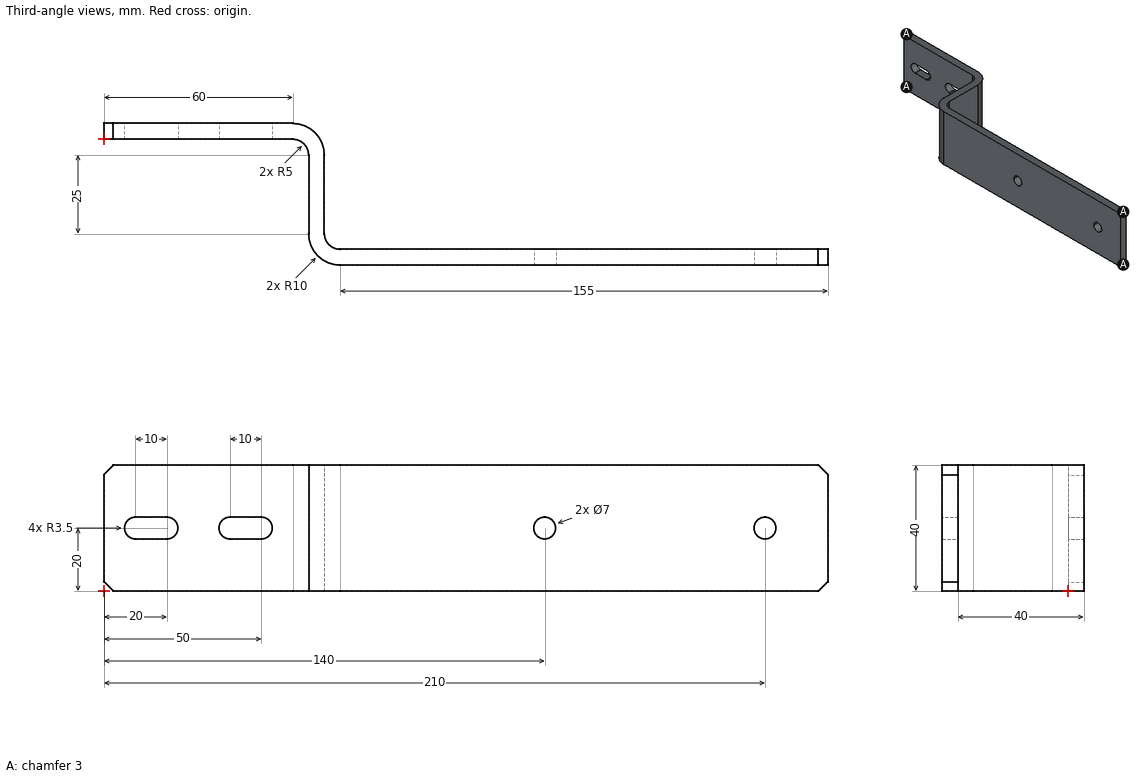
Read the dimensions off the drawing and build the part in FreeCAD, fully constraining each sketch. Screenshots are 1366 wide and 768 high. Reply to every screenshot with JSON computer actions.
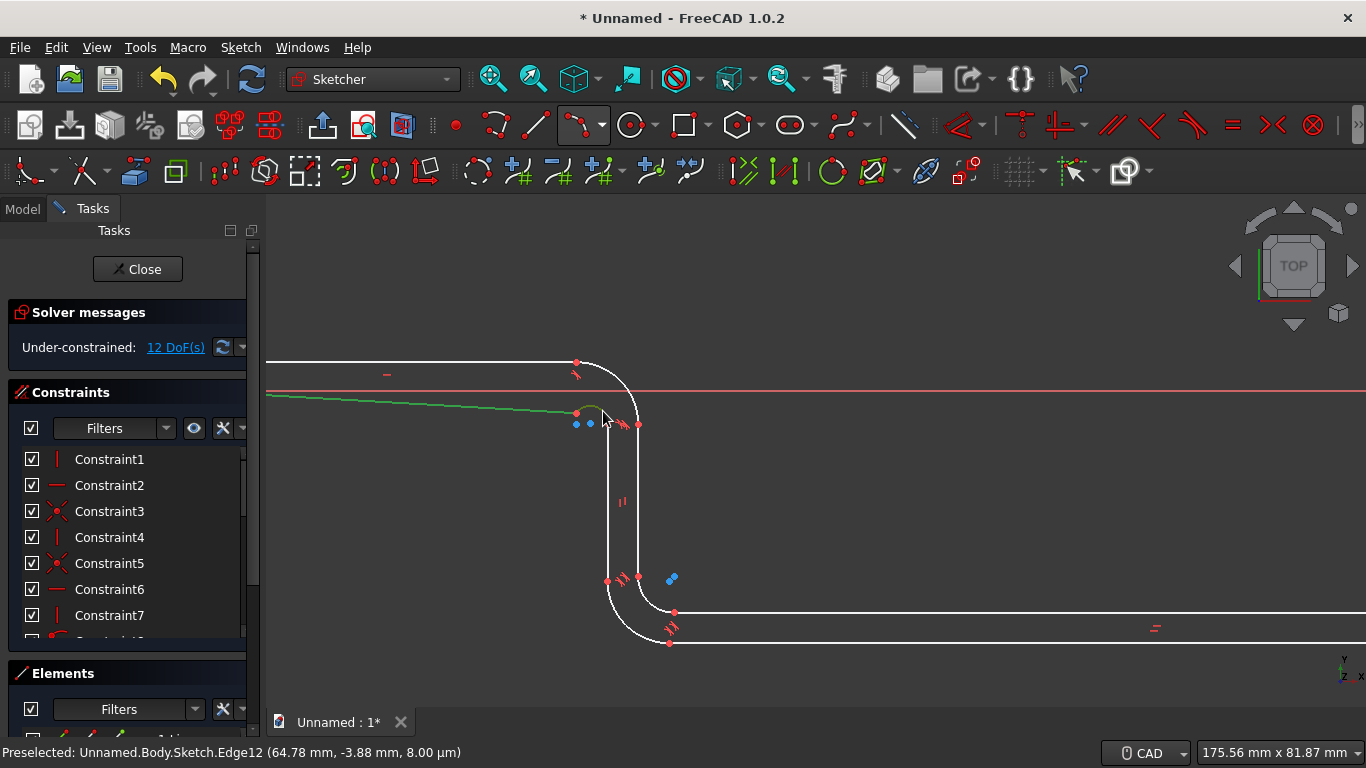
{"action": "left_click", "coordinate": [1194, 126]}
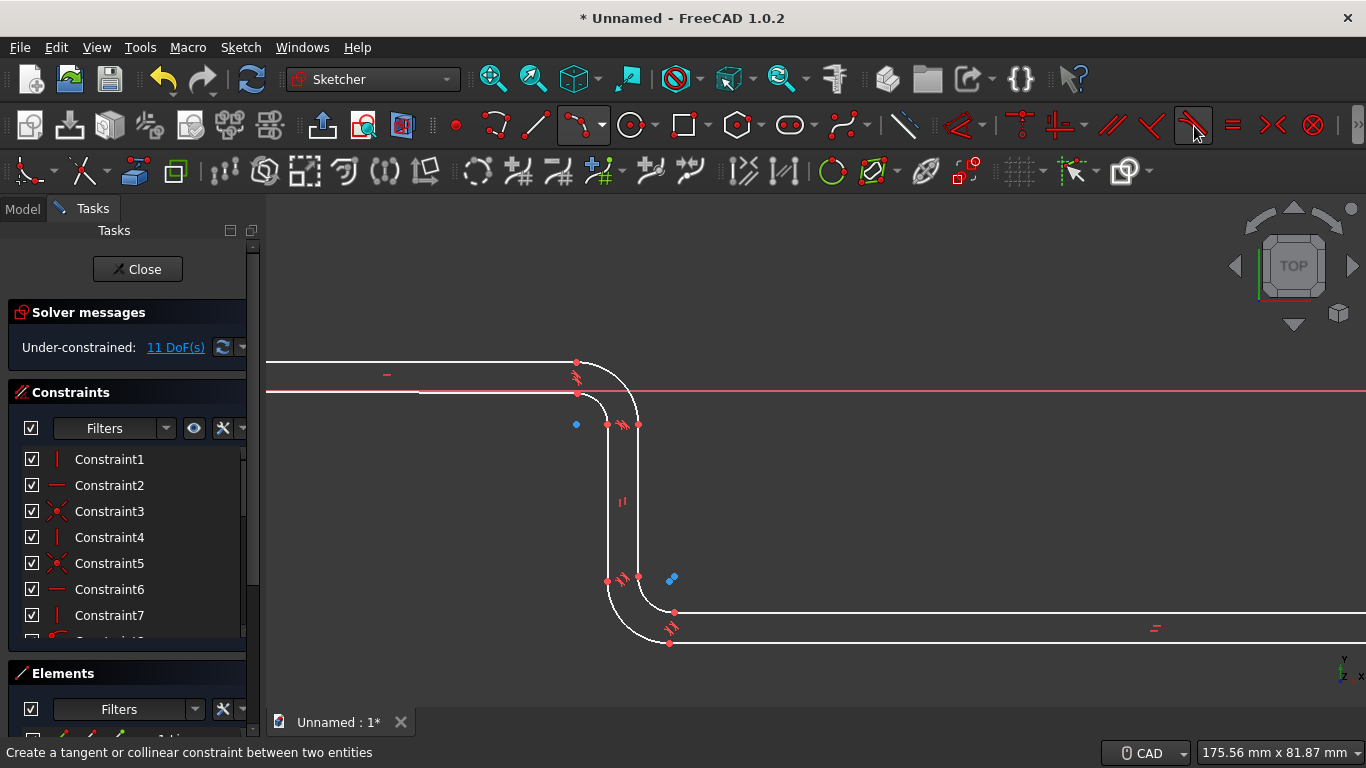
{"action": "left_click", "coordinate": [313, 392]}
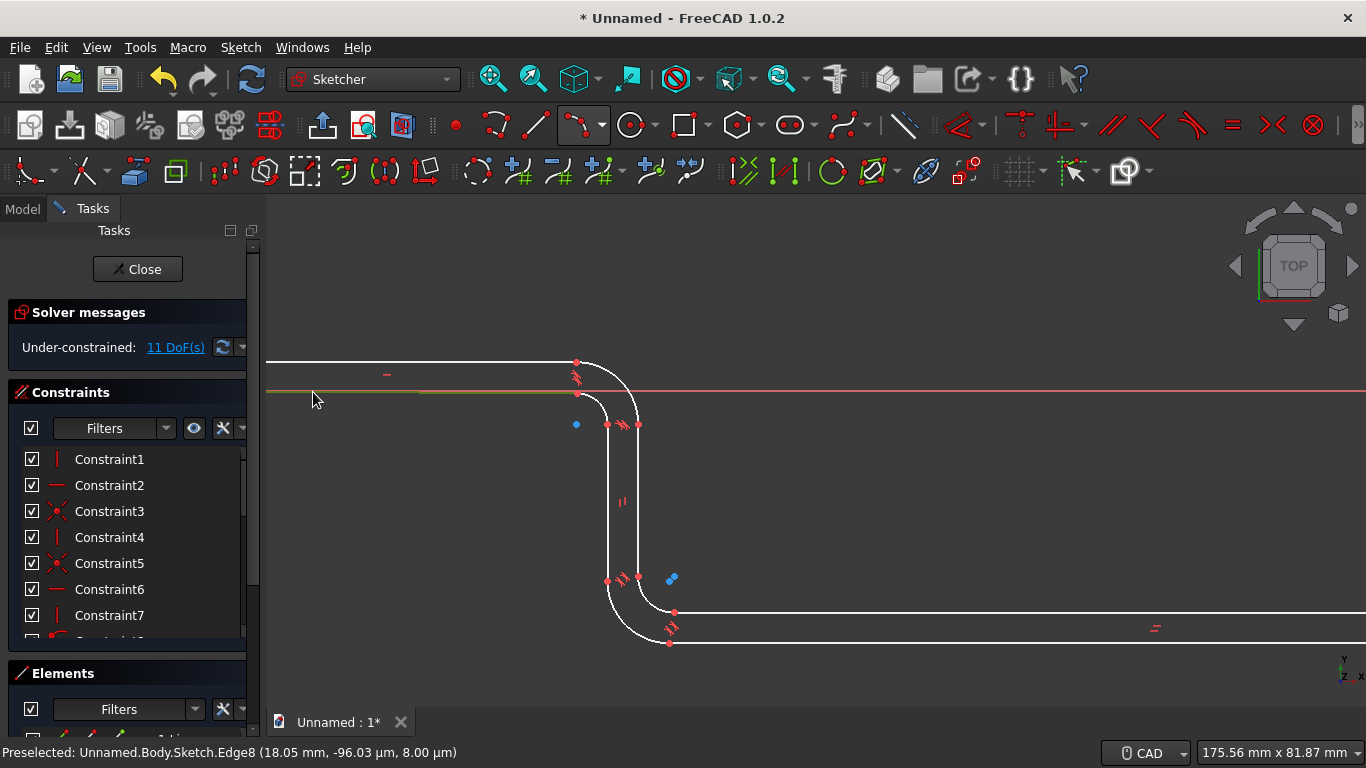
{"action": "key", "text": "h"}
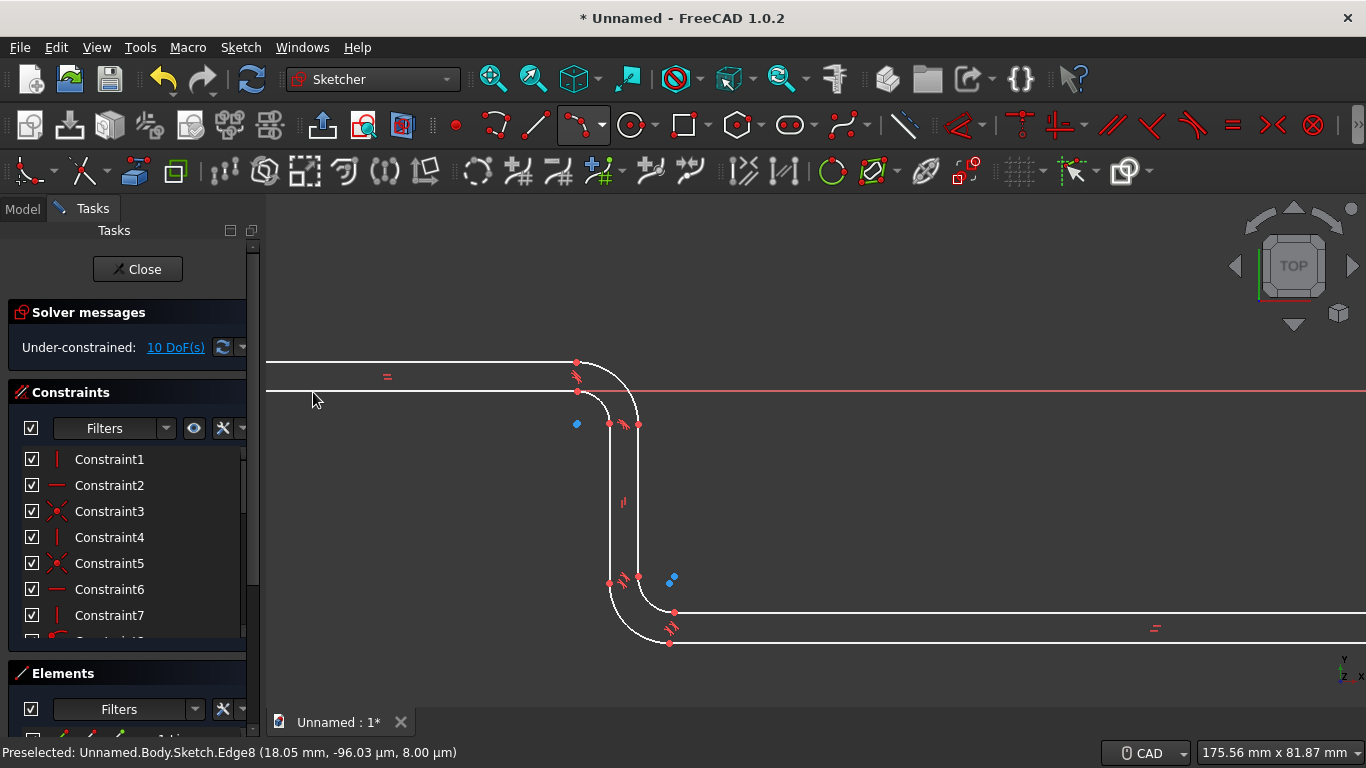
{"action": "left_click", "coordinate": [616, 610]}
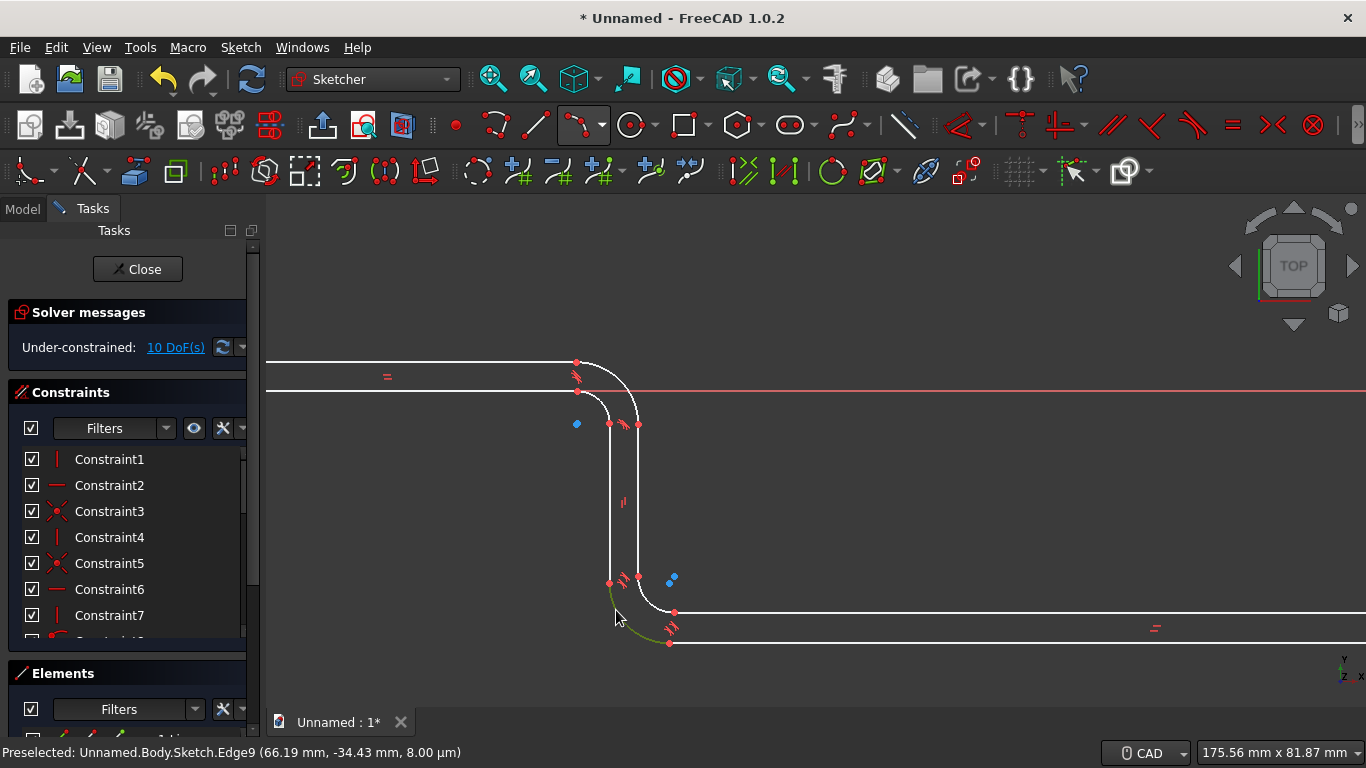
{"action": "left_click", "coordinate": [642, 593]}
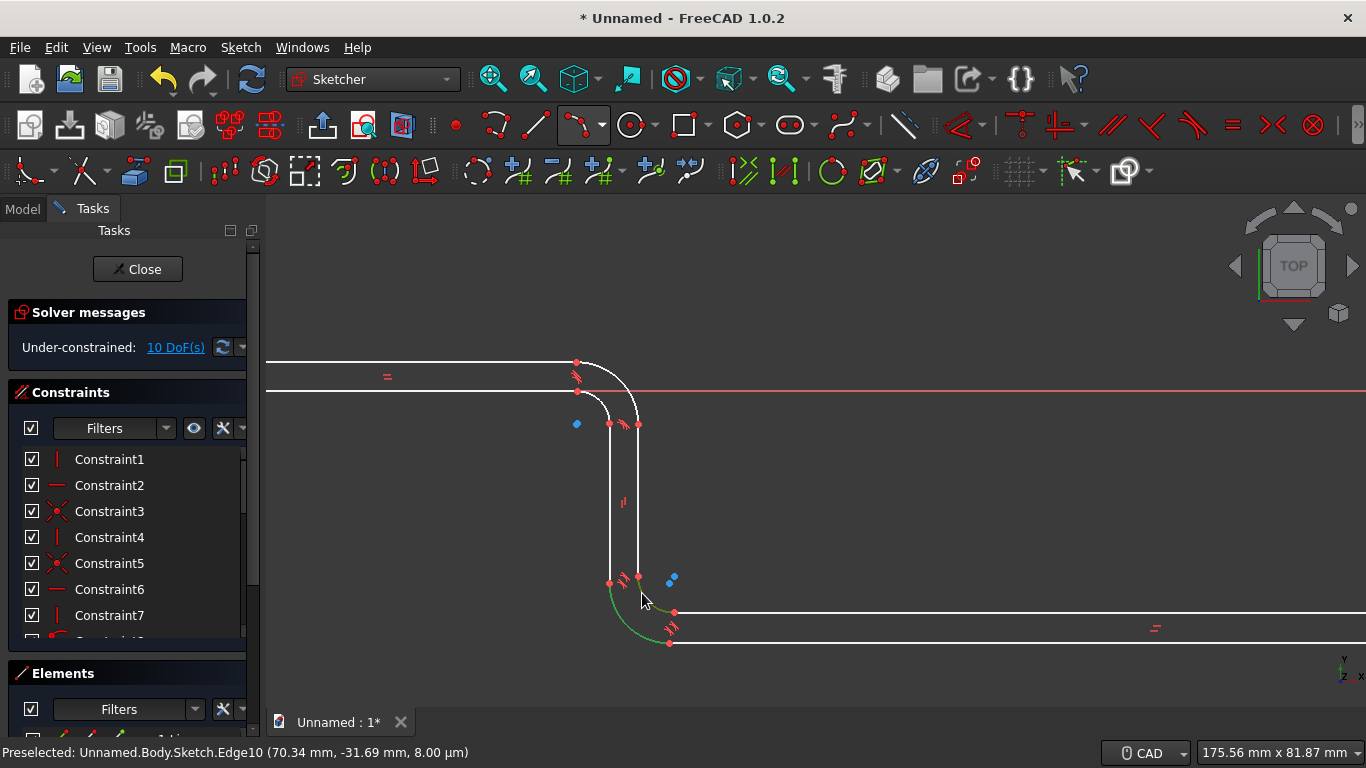
{"action": "left_click", "coordinate": [1020, 126]}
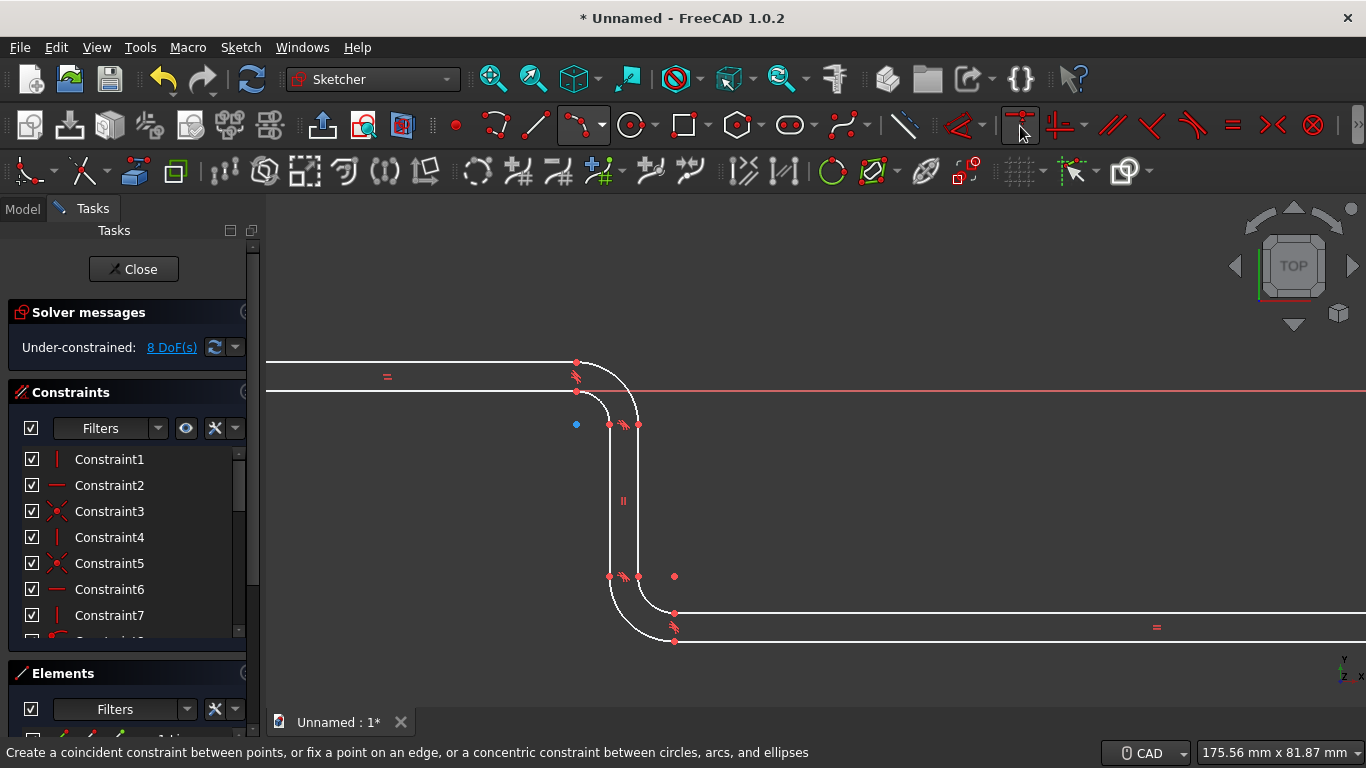
{"action": "left_click", "coordinate": [604, 369]}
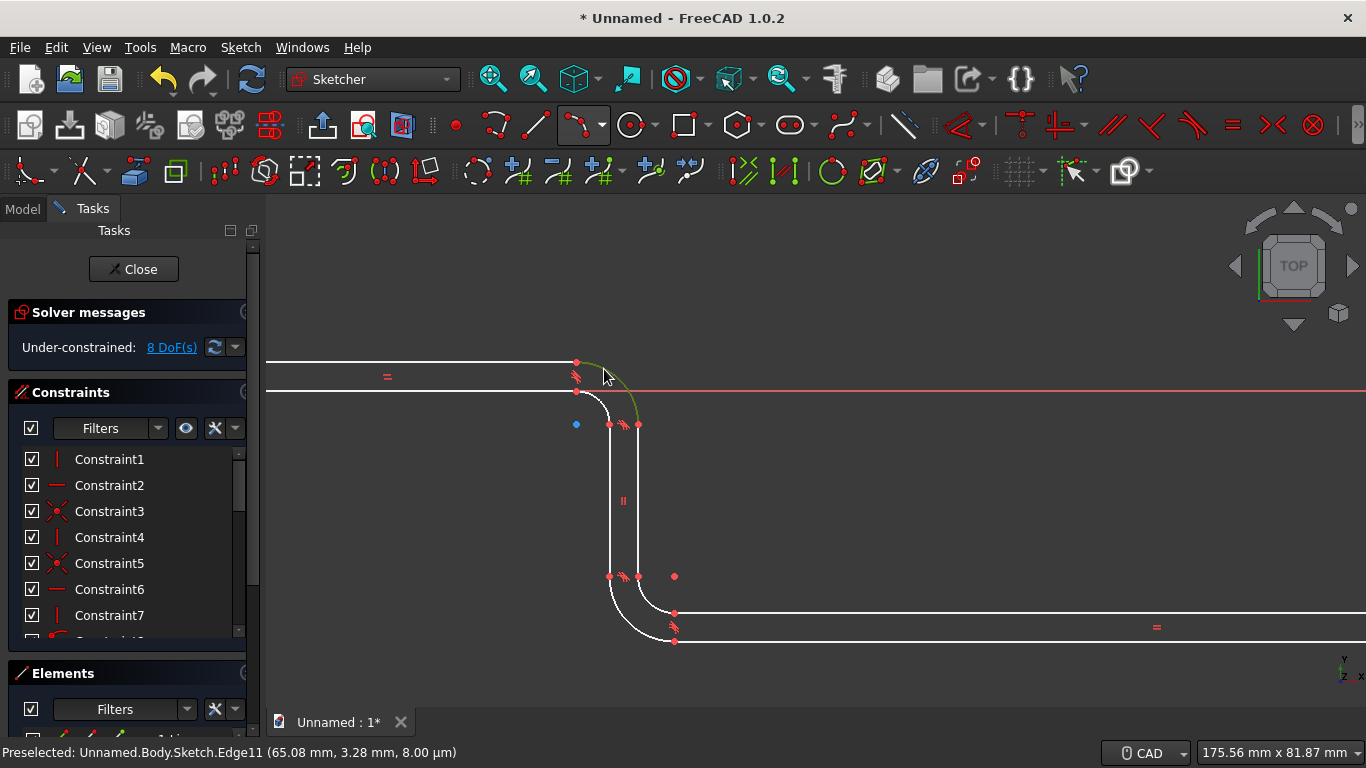
{"action": "left_click", "coordinate": [606, 409]}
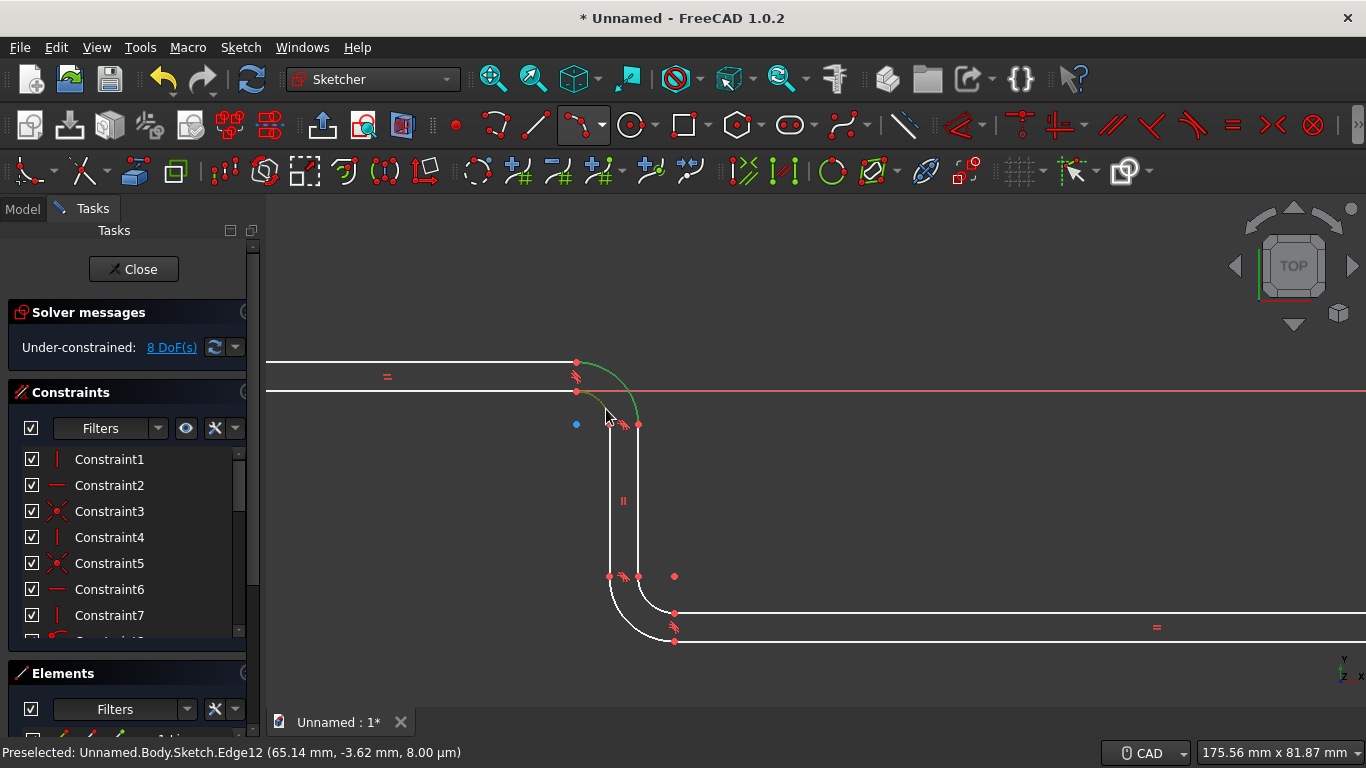
{"action": "left_click", "coordinate": [1020, 126]}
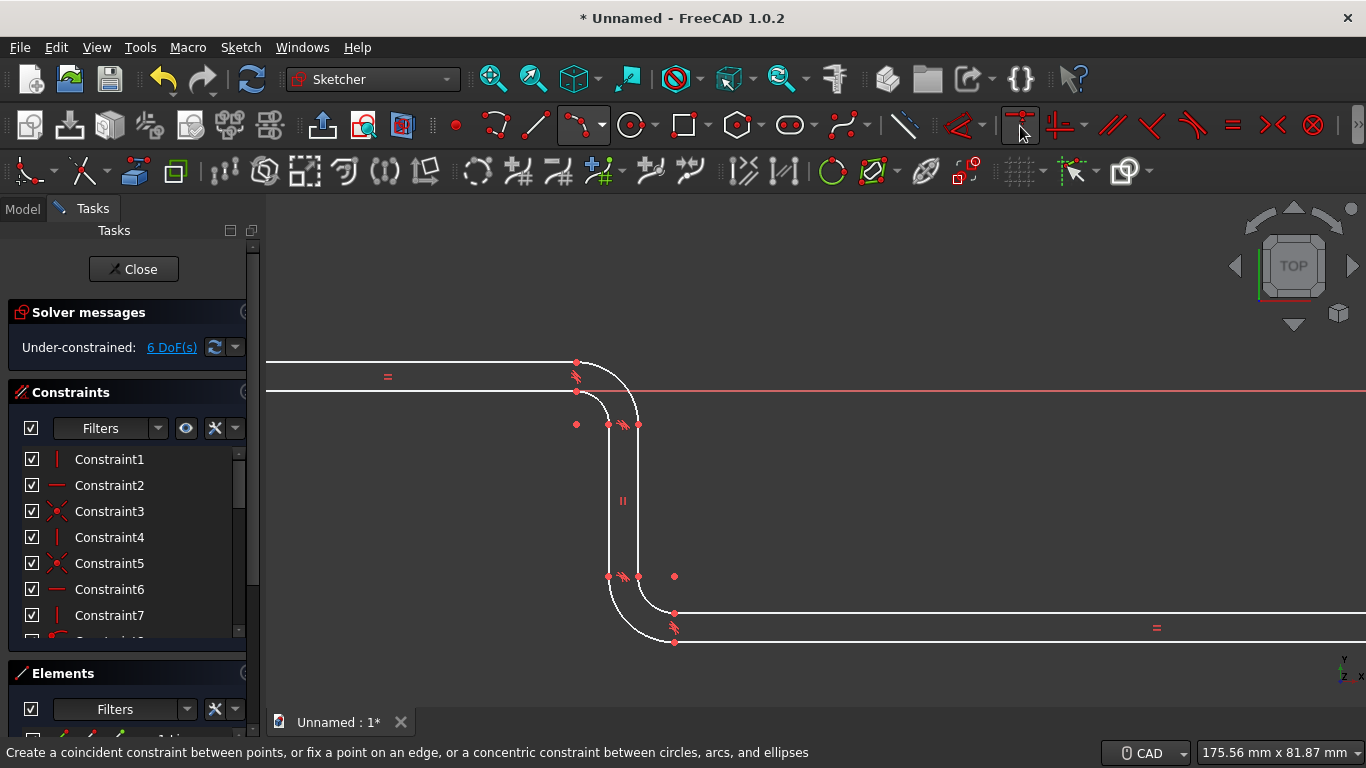
{"action": "left_click", "coordinate": [616, 607]}